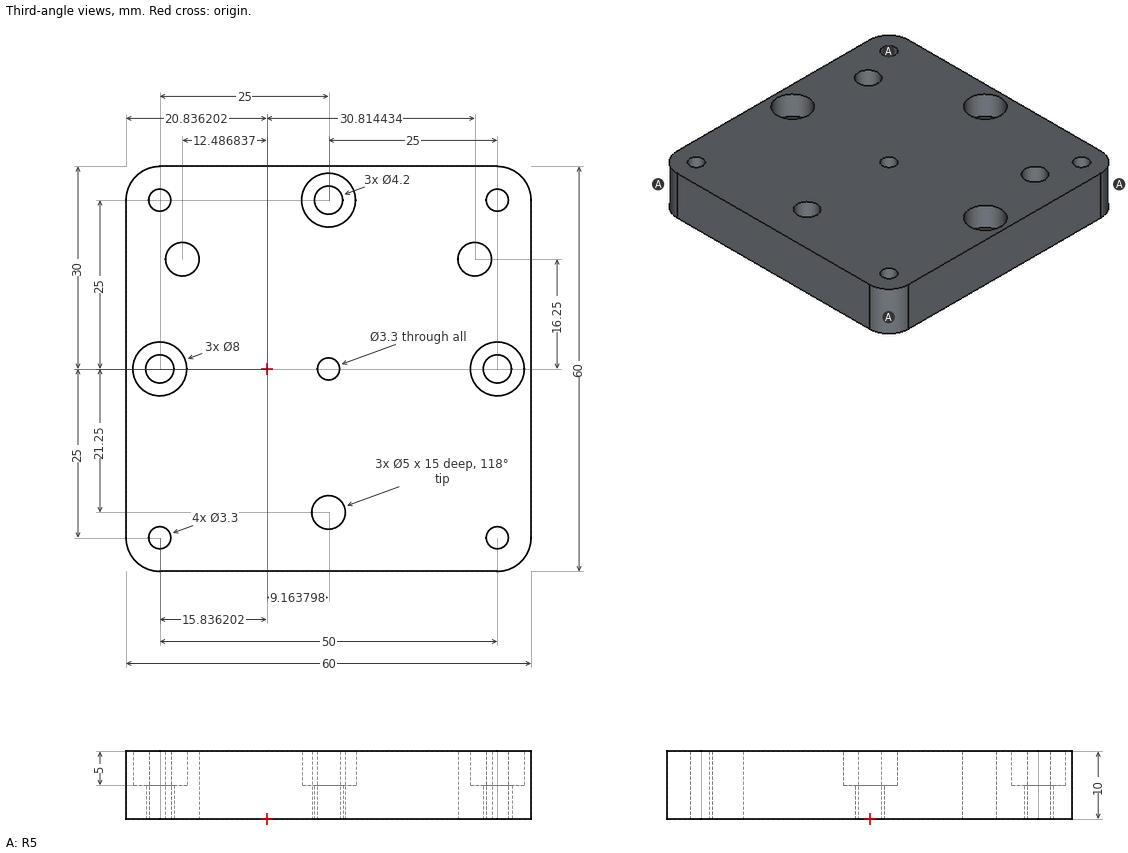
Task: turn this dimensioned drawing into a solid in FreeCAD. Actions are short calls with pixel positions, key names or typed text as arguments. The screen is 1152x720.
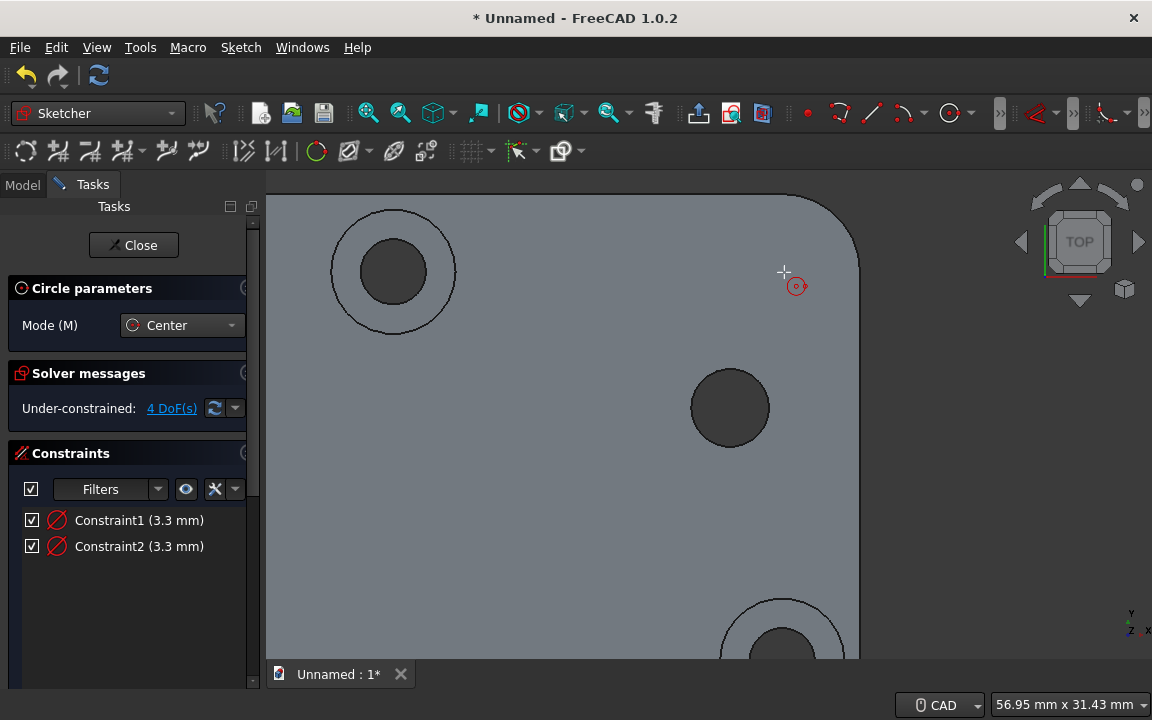
click(782, 272)
move(800, 254)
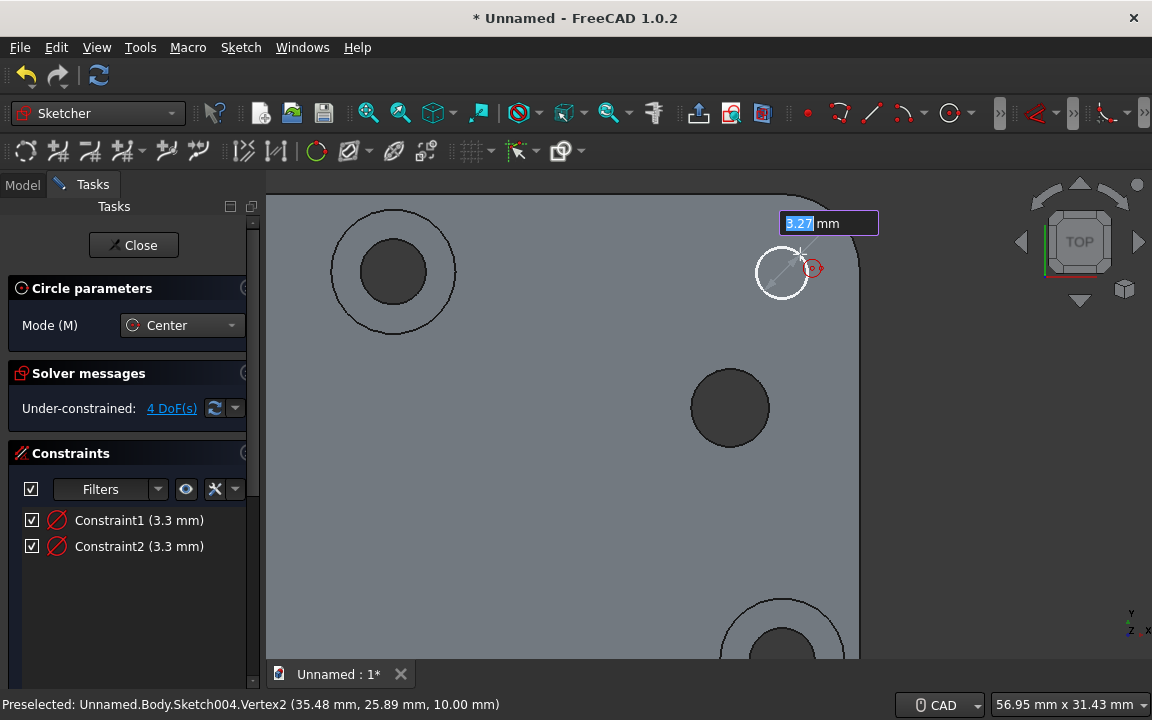
text(3.3)
key(Return)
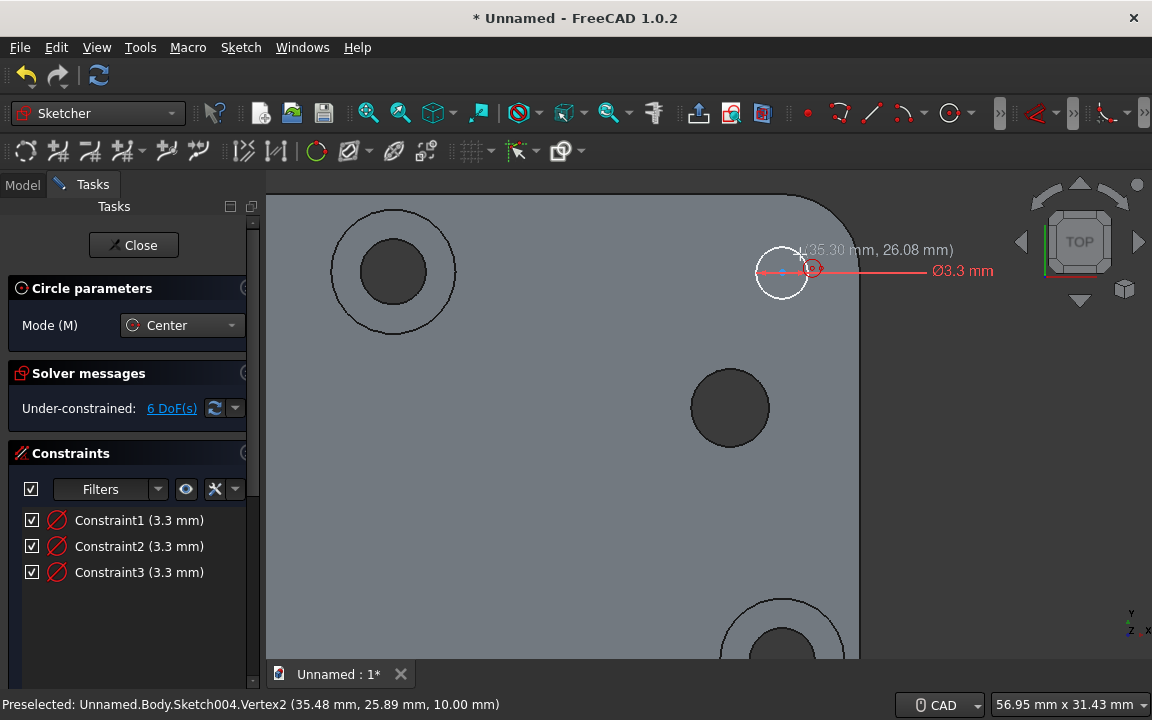
scroll(784, 271, down, 5)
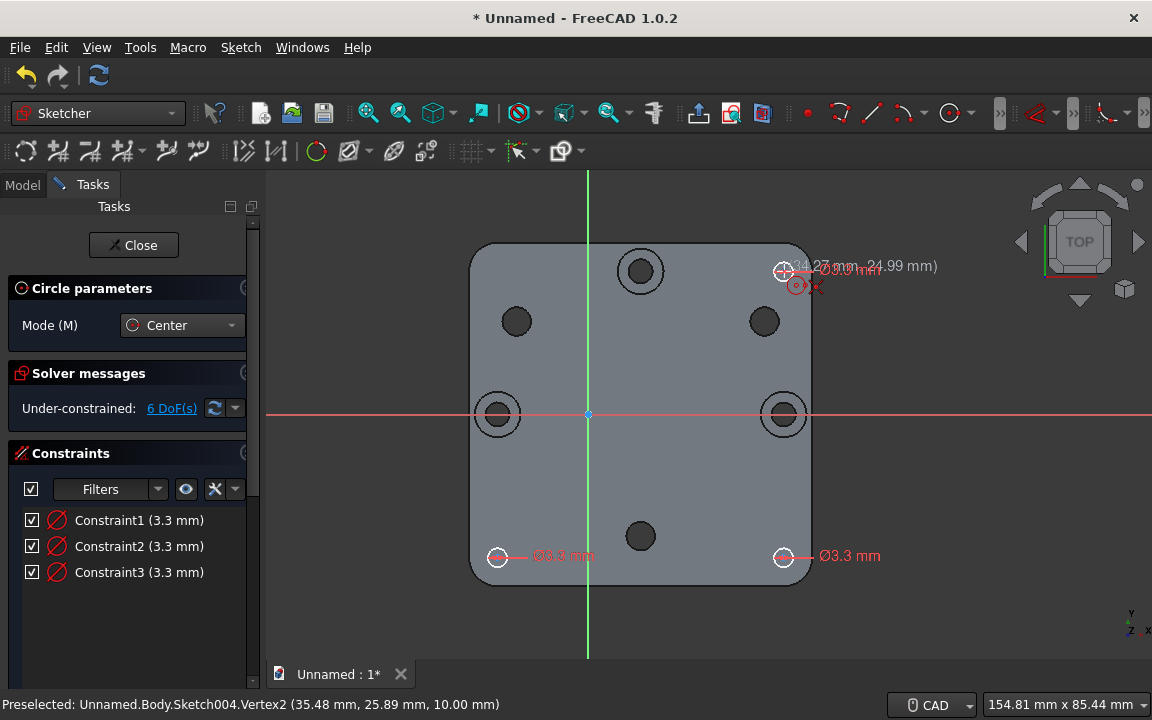
scroll(498, 271, up, 5)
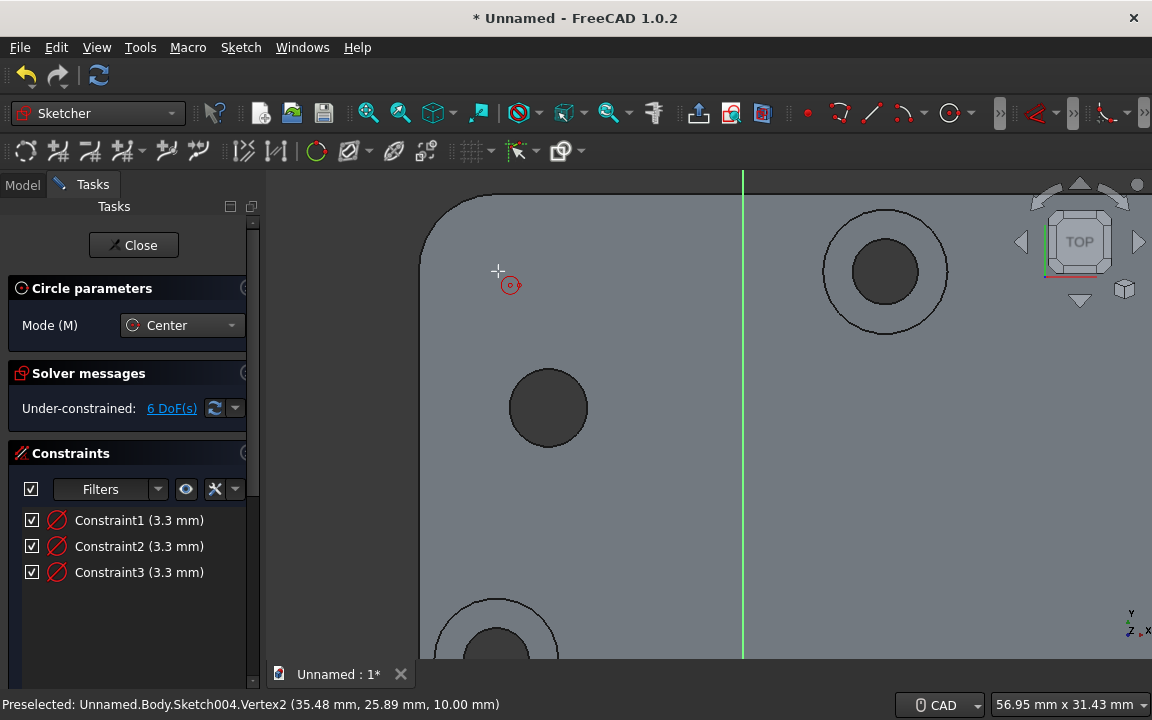
click(496, 272)
move(515, 254)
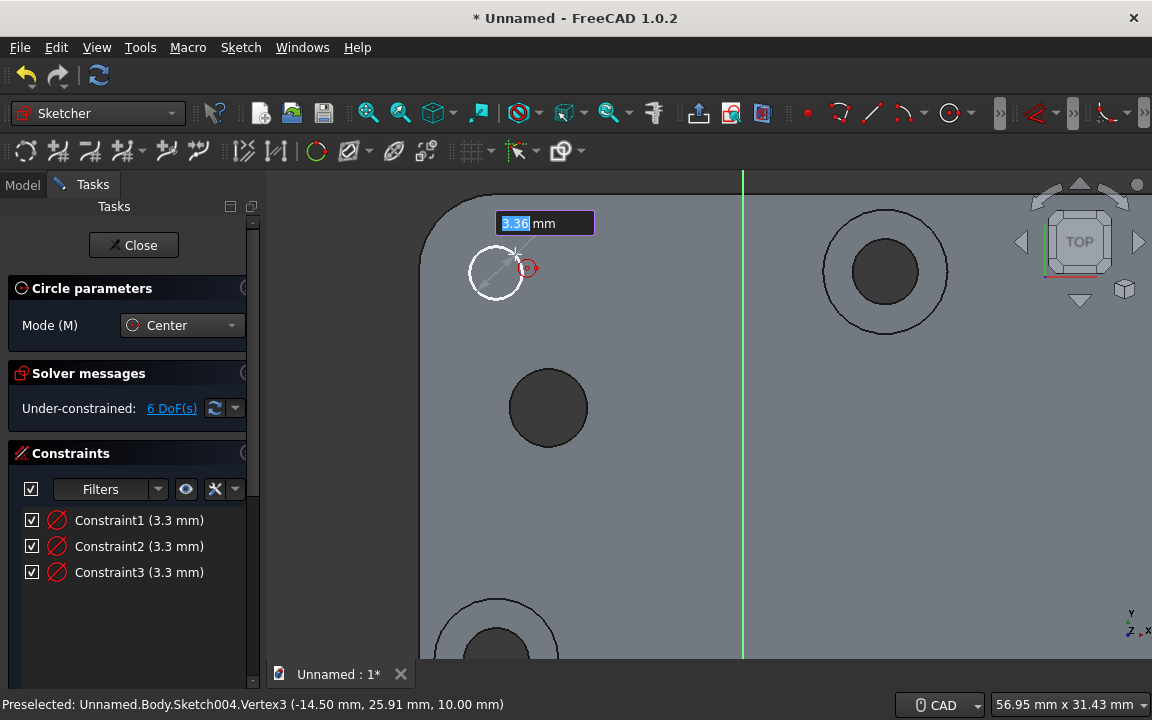
text(3.3)
key(Return)
key(Escape)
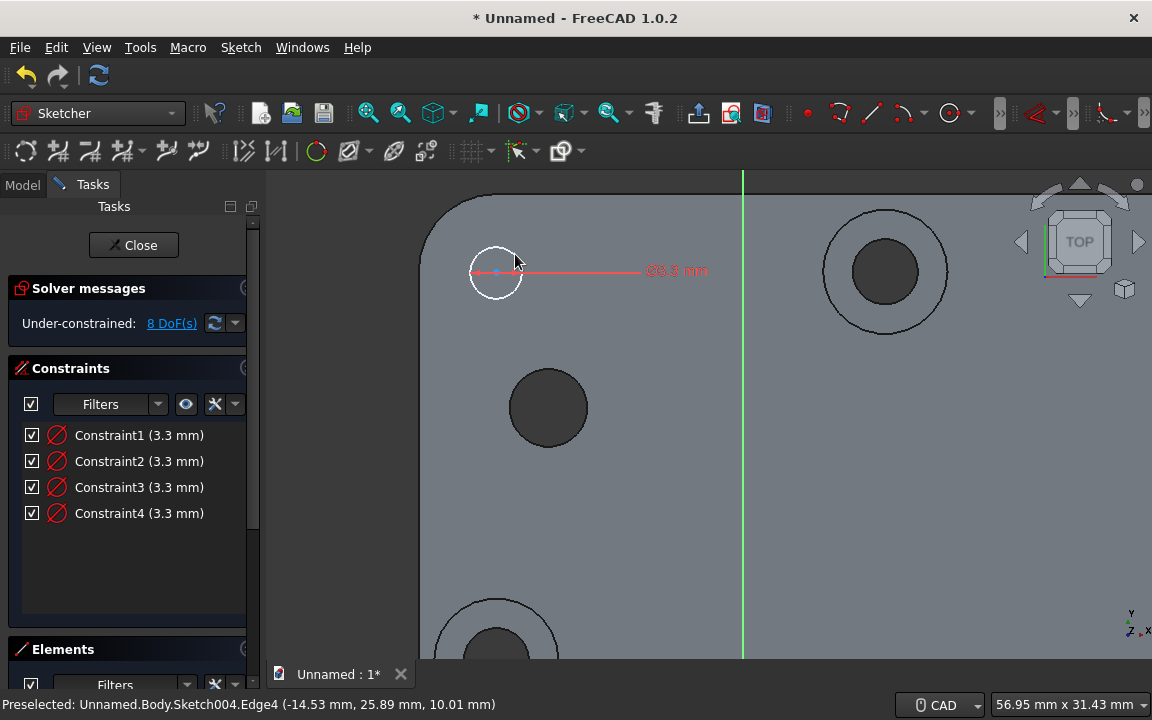
scroll(498, 271, down, 5)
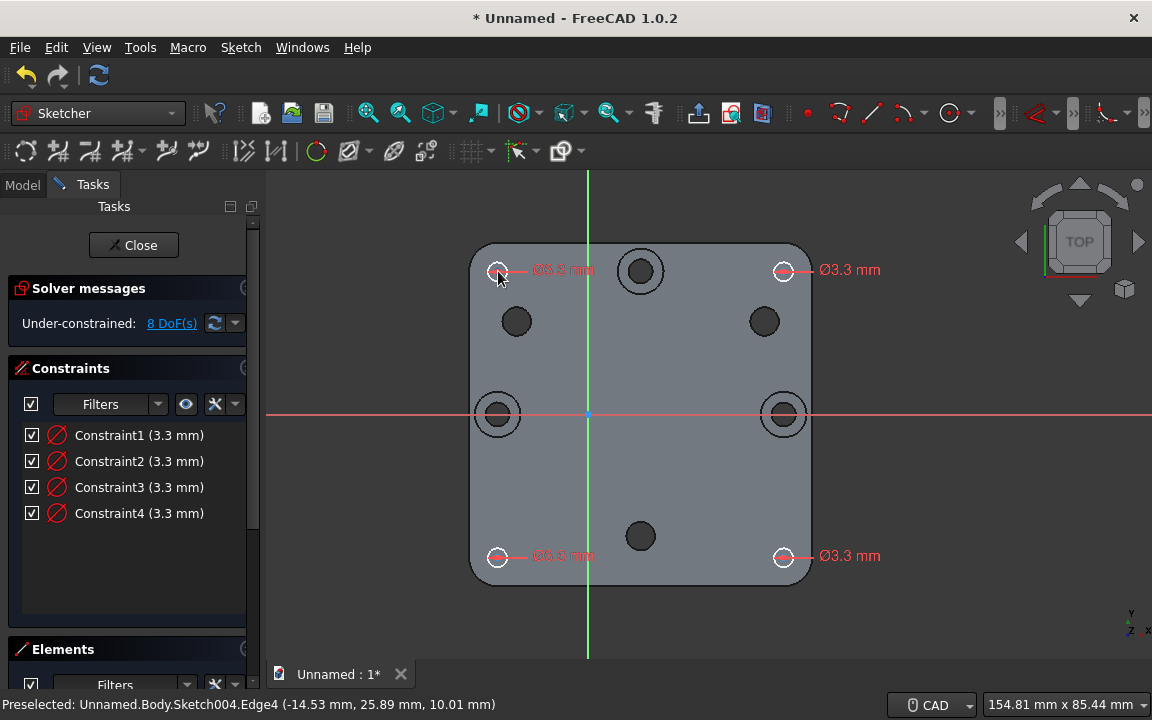
click(498, 558)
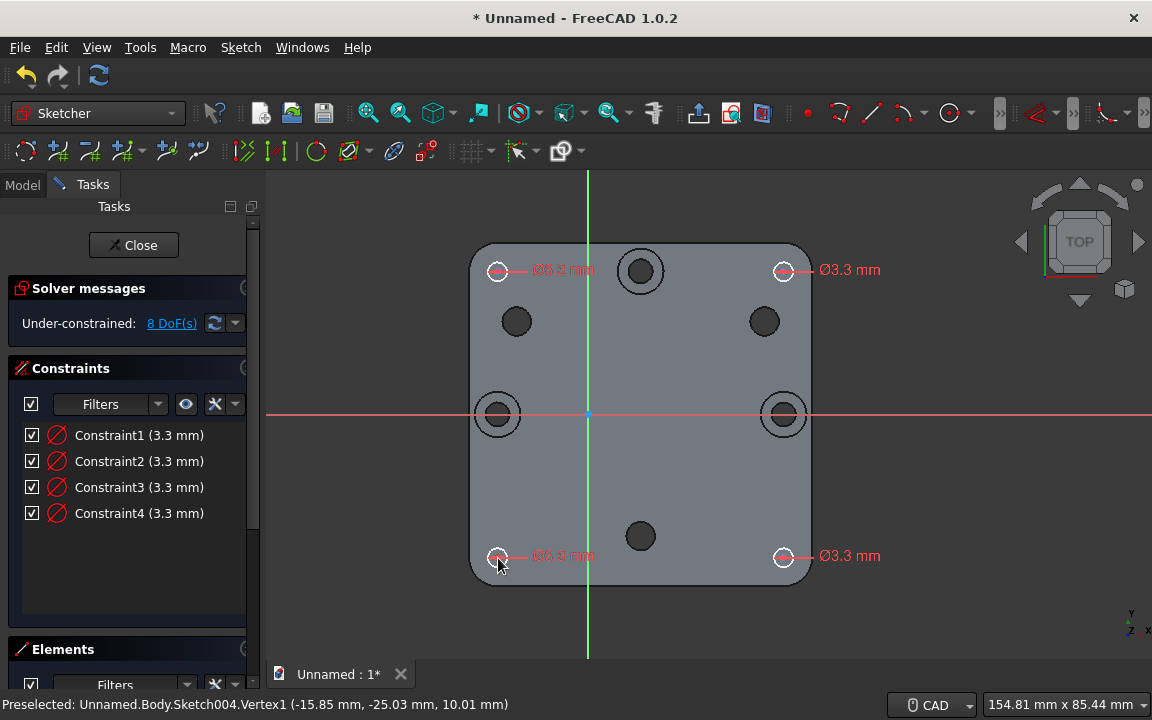
click(784, 558)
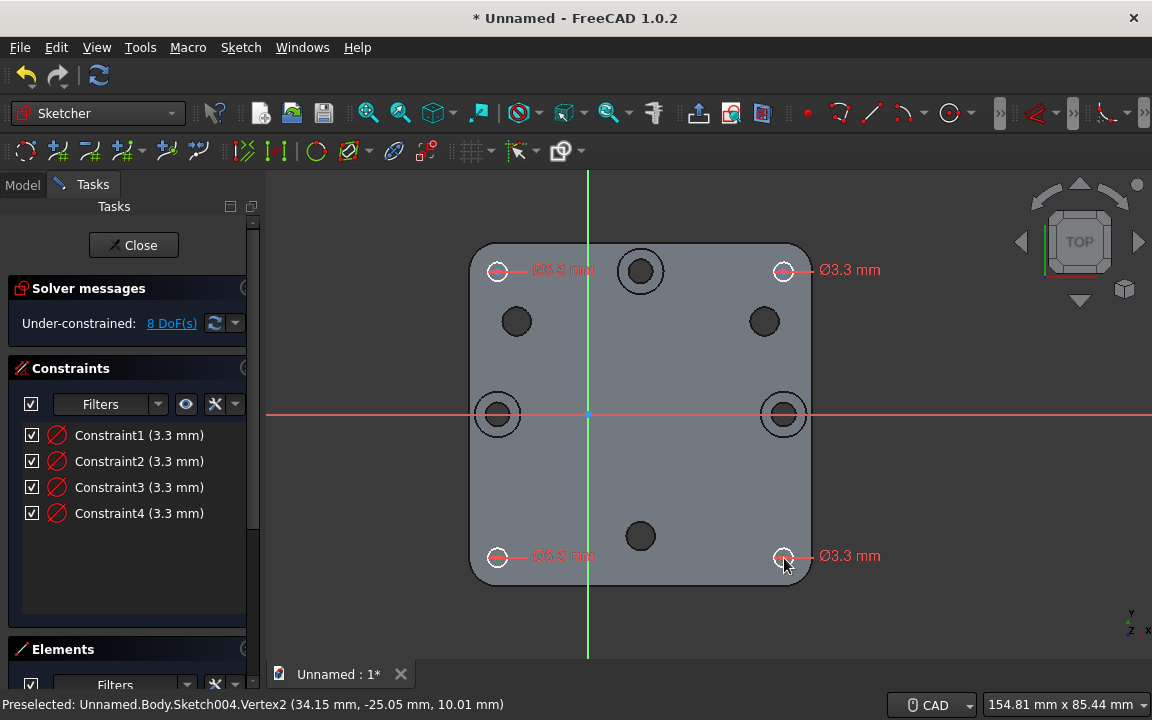
key(h)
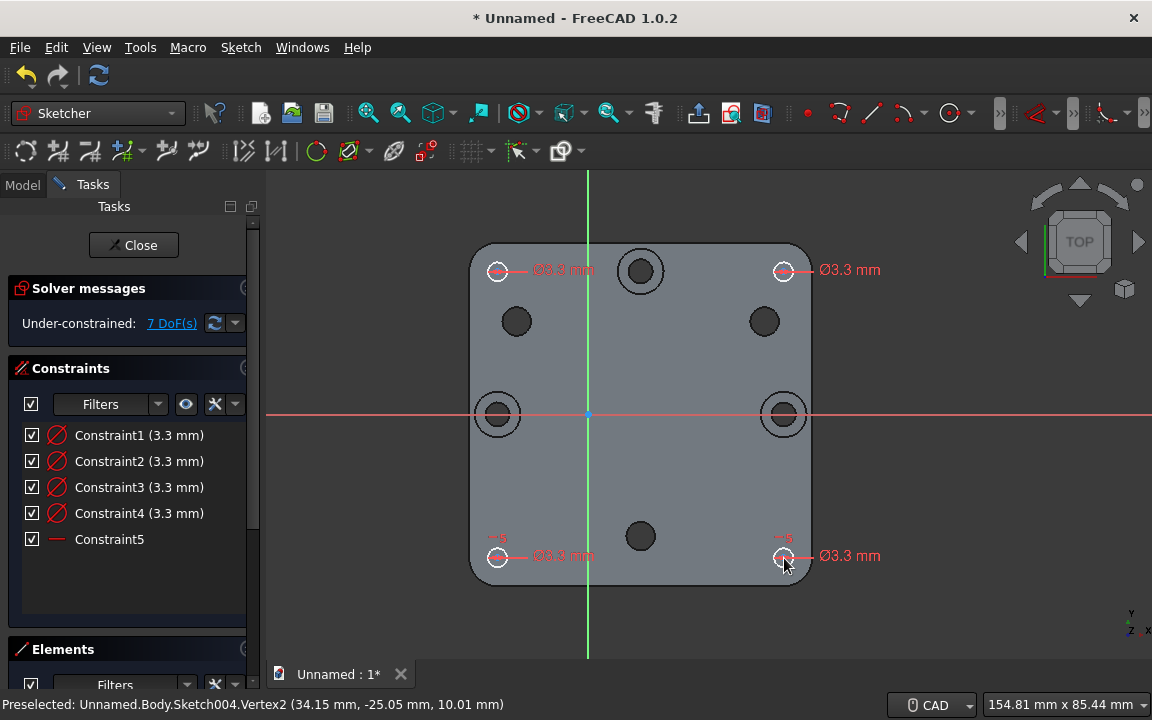
click(784, 558)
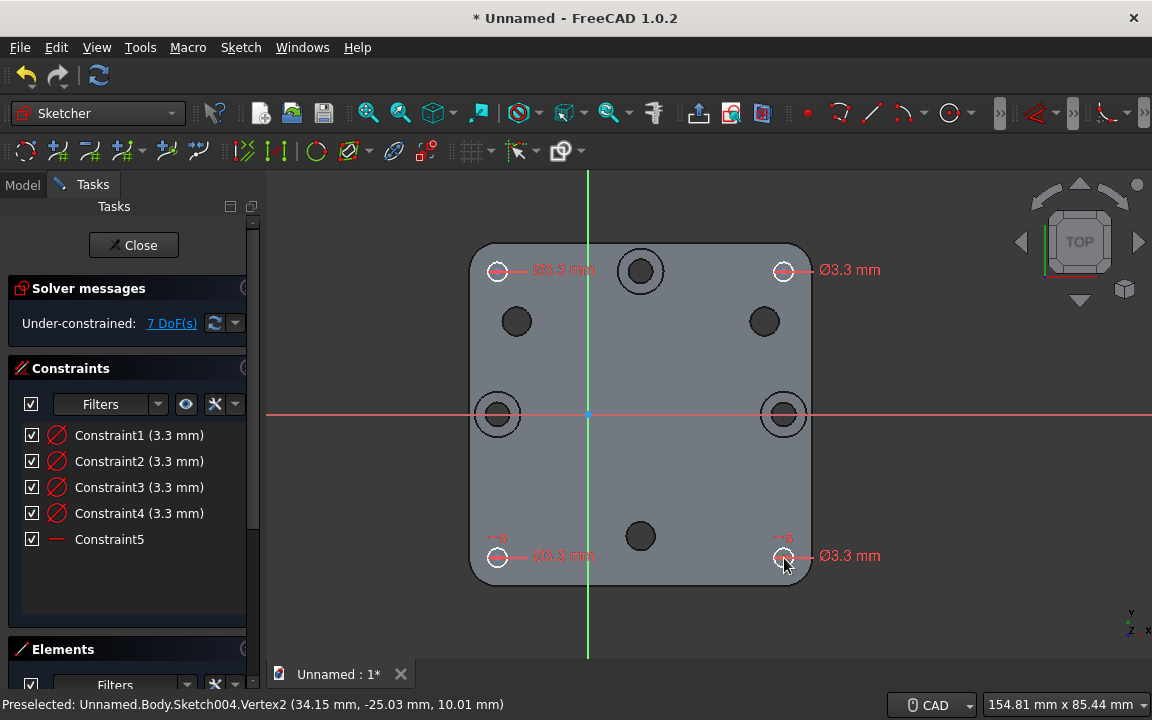
click(784, 272)